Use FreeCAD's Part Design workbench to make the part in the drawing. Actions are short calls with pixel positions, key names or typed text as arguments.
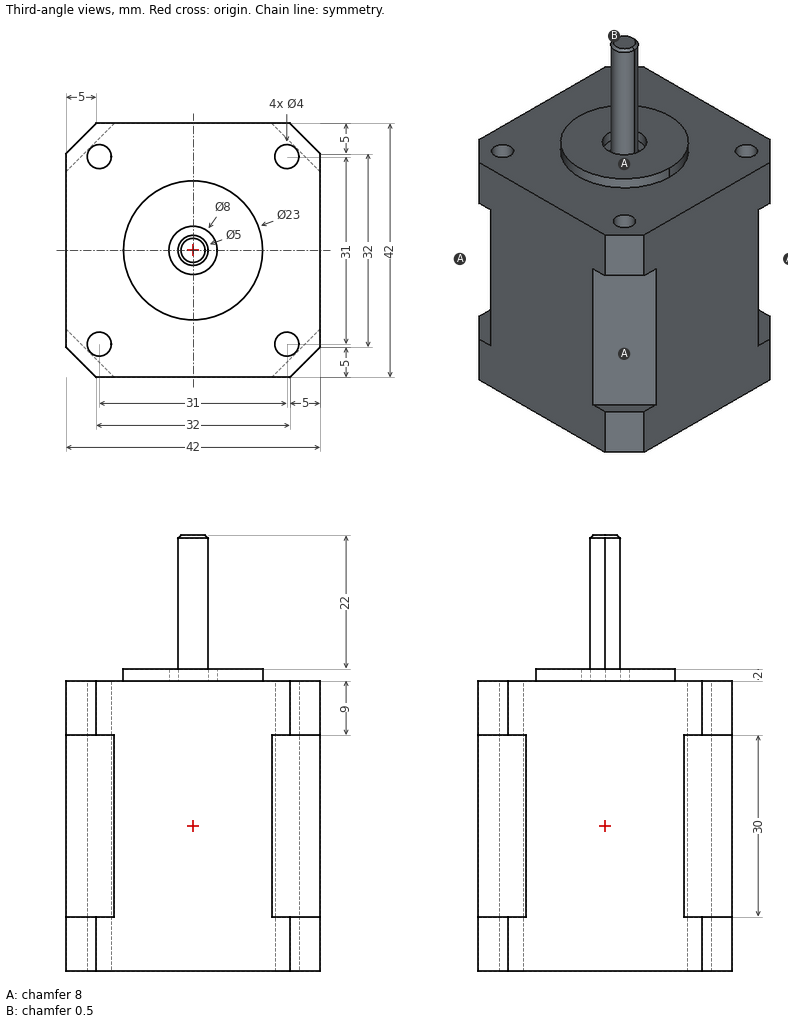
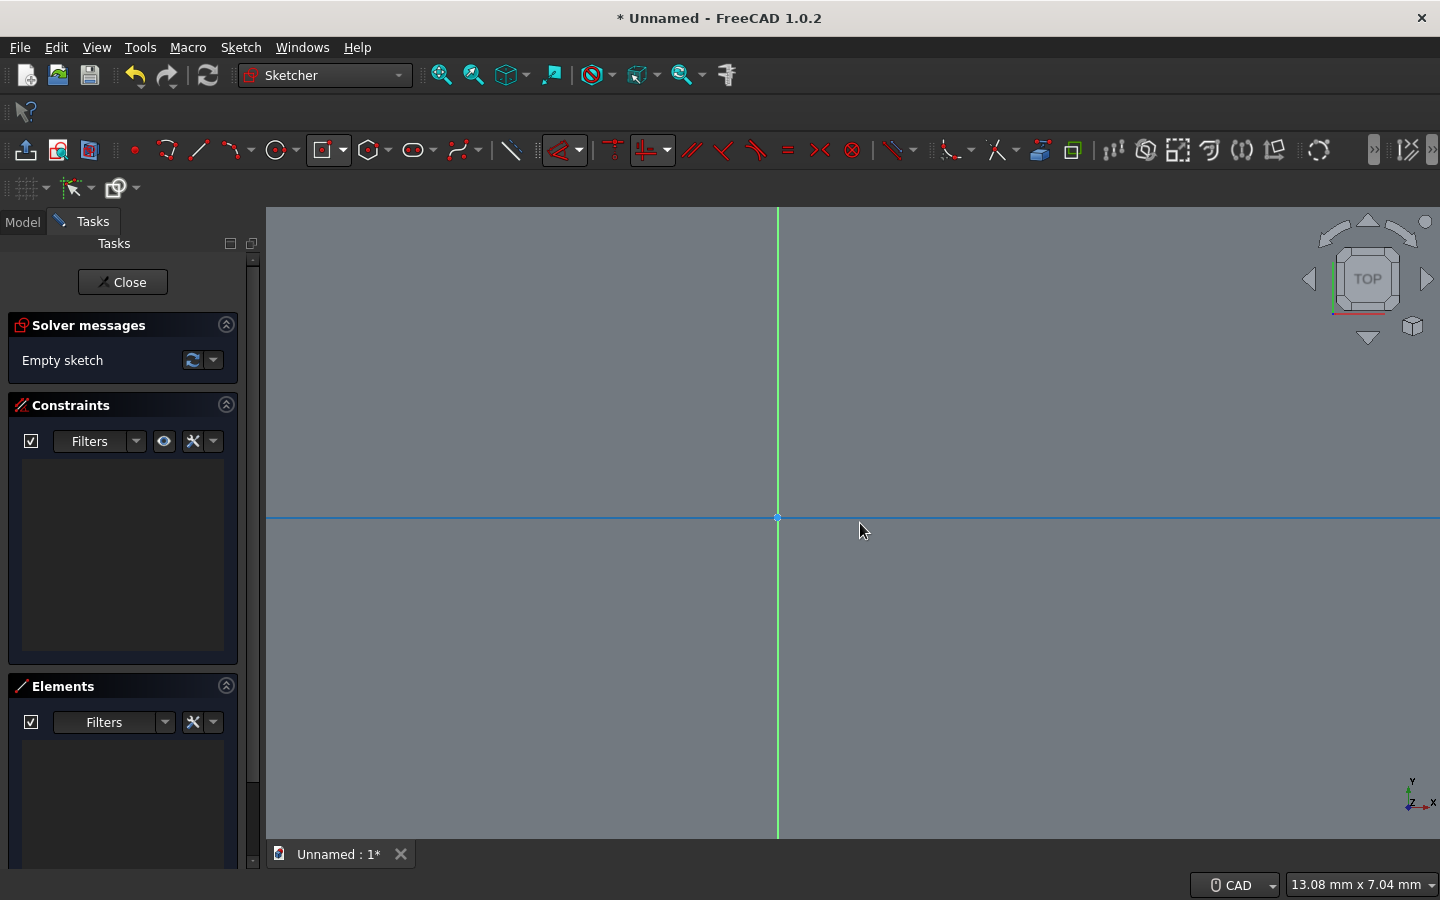
click(276, 150)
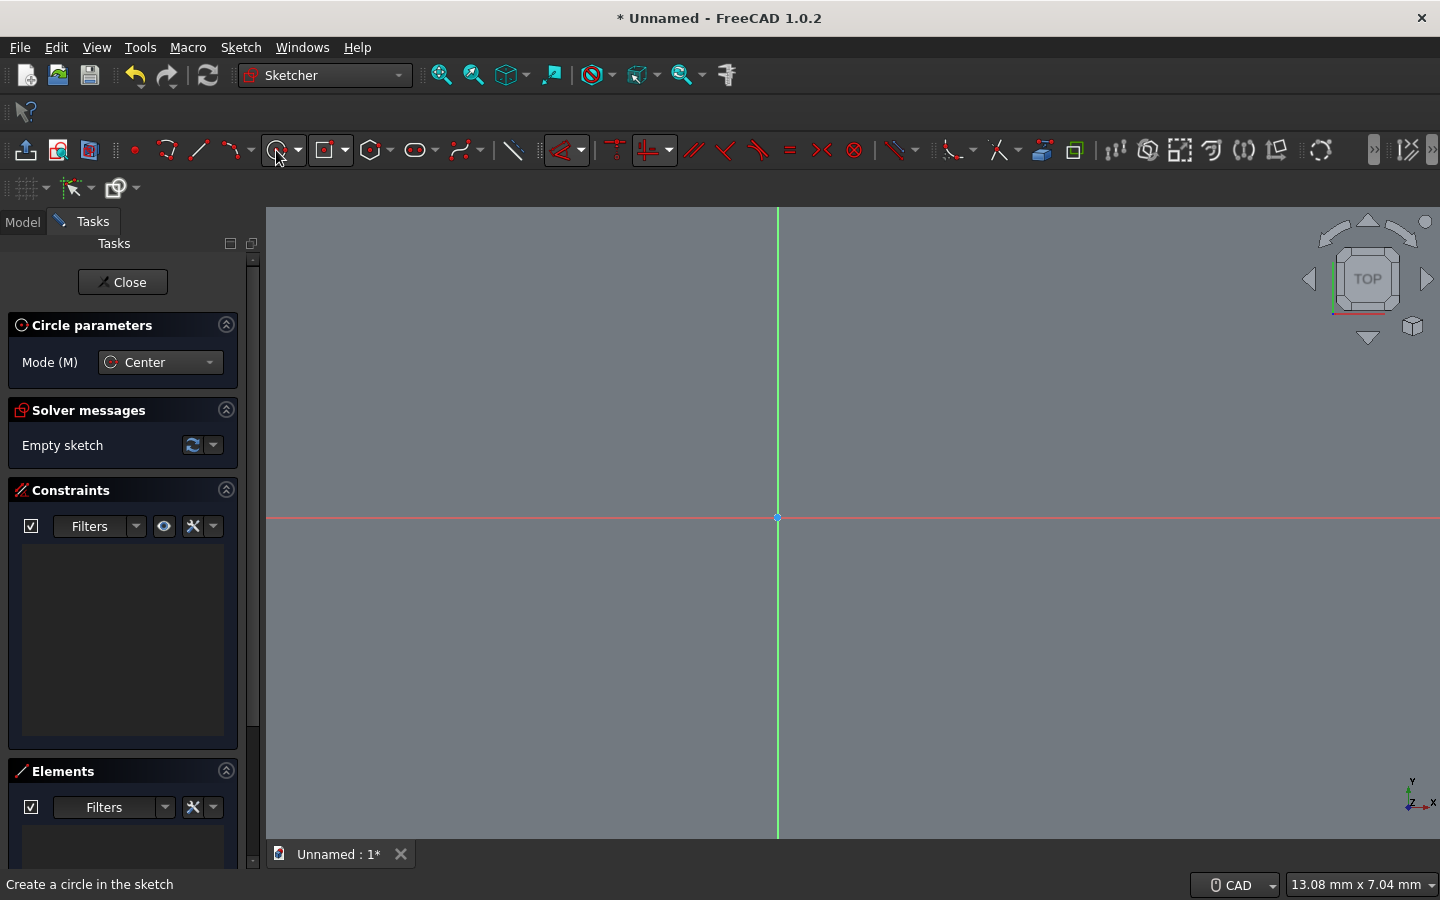
click(778, 518)
move(936, 359)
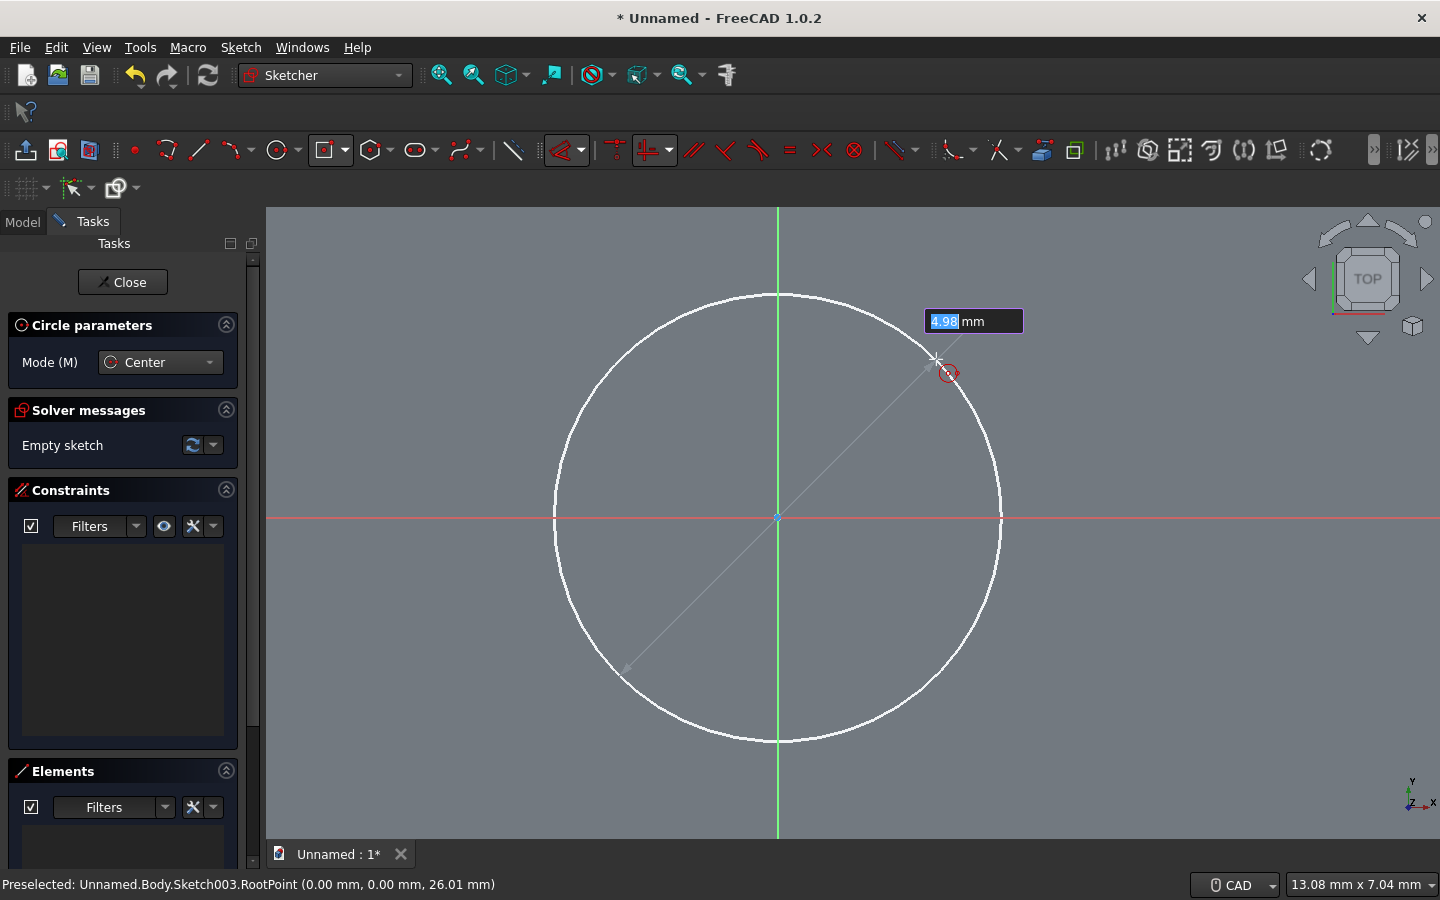
text(5)
key(Return)
key(Escape)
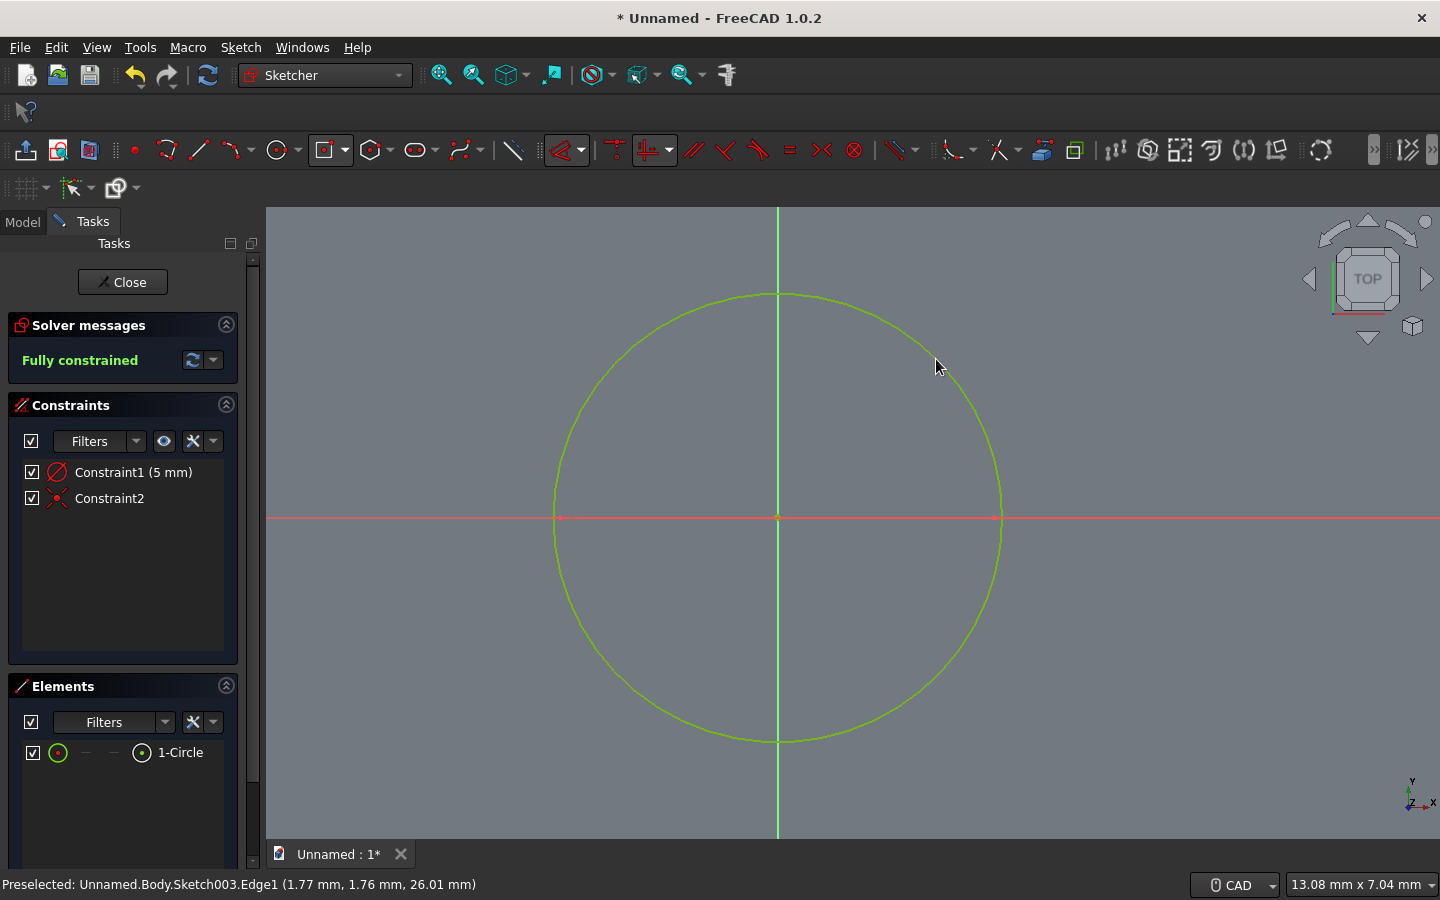
click(123, 282)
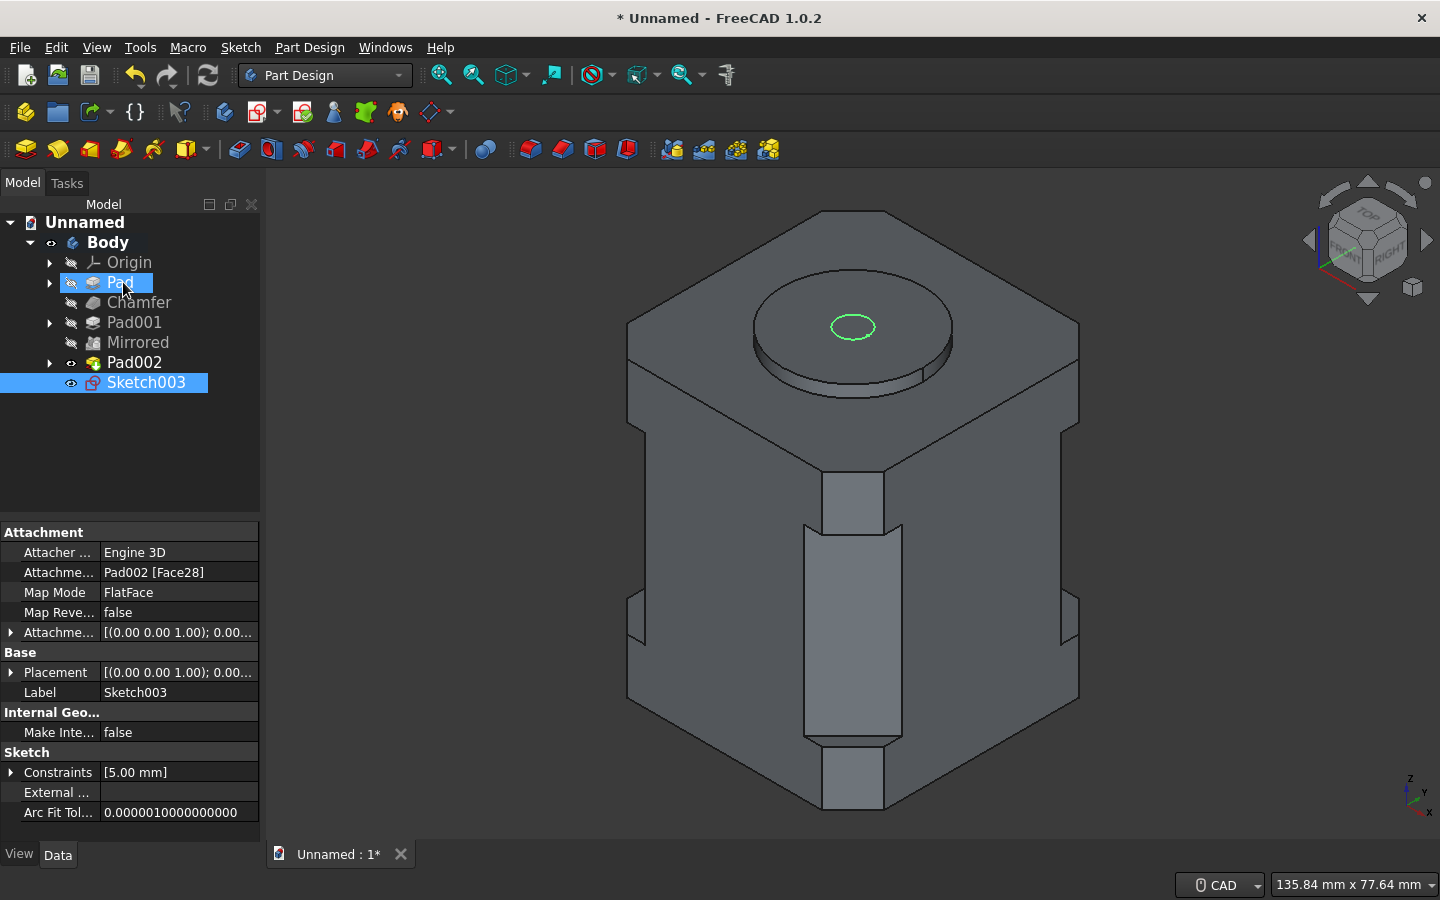
click(26, 150)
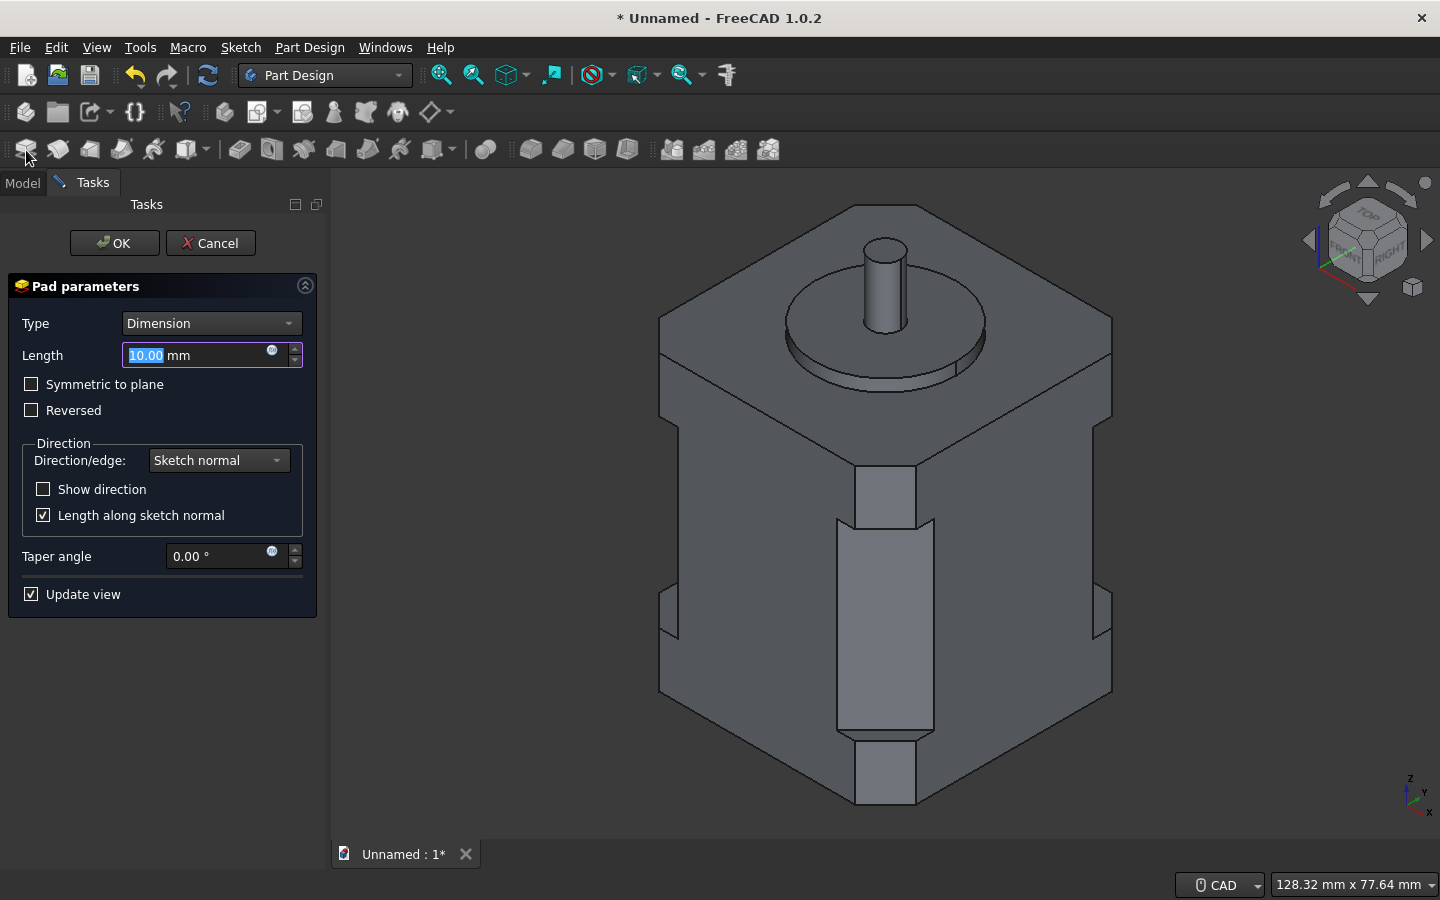
text(22)
key(Tab)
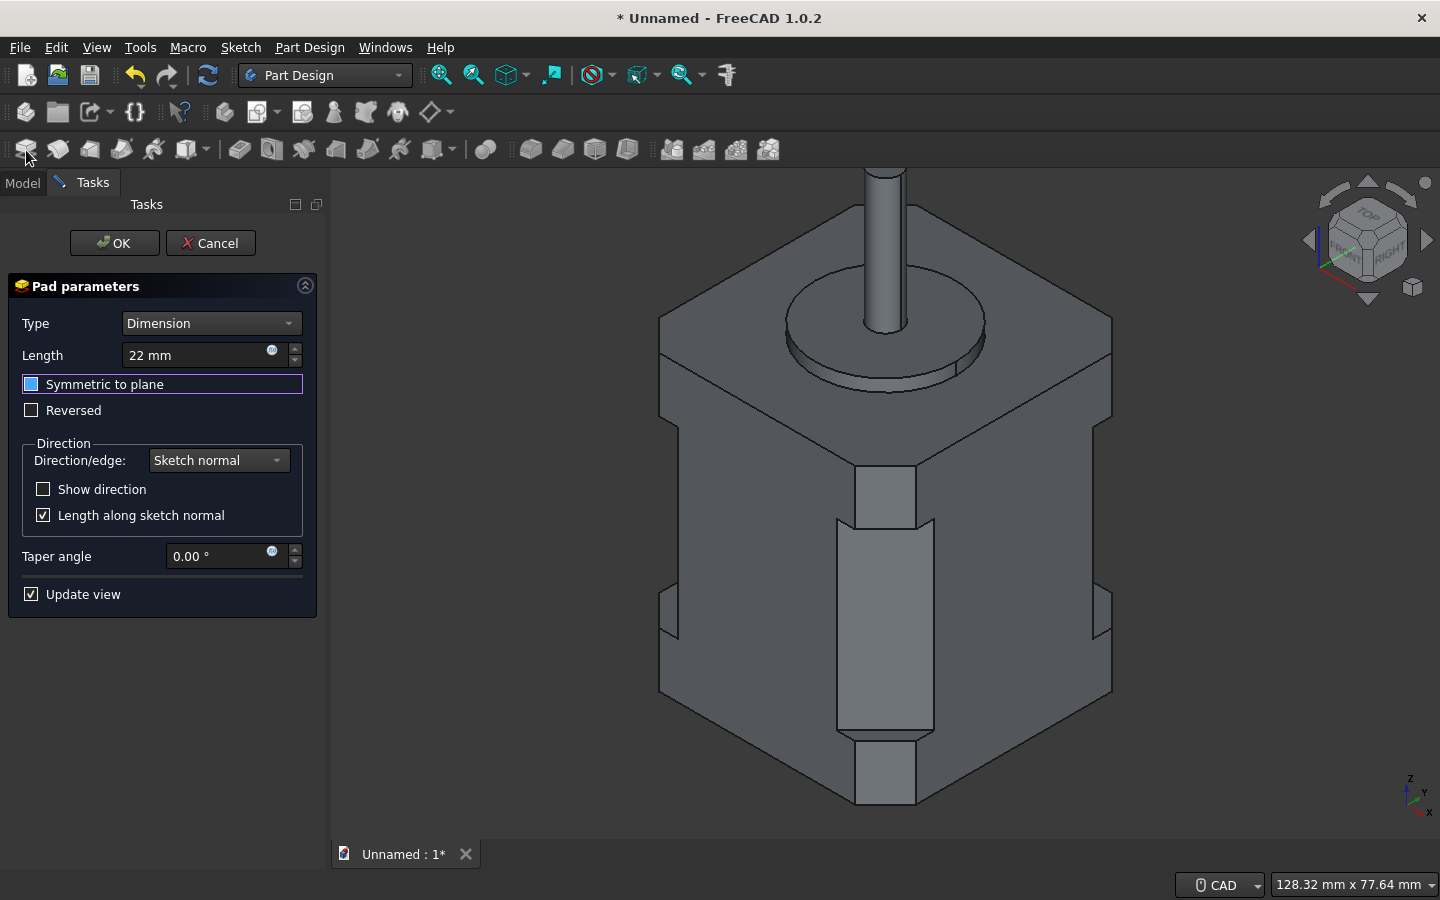
click(115, 243)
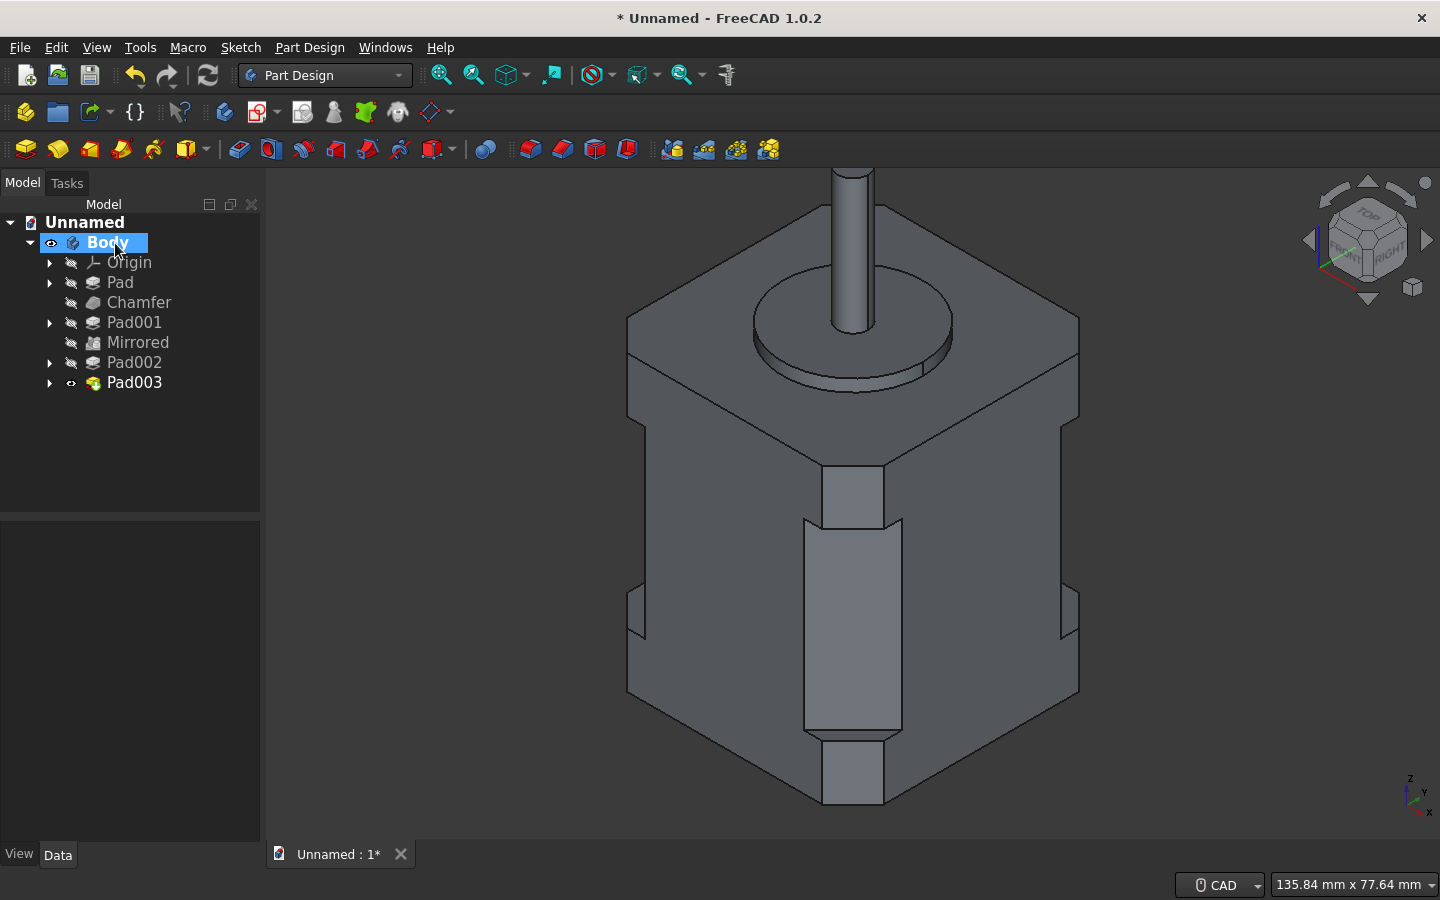
click(442, 76)